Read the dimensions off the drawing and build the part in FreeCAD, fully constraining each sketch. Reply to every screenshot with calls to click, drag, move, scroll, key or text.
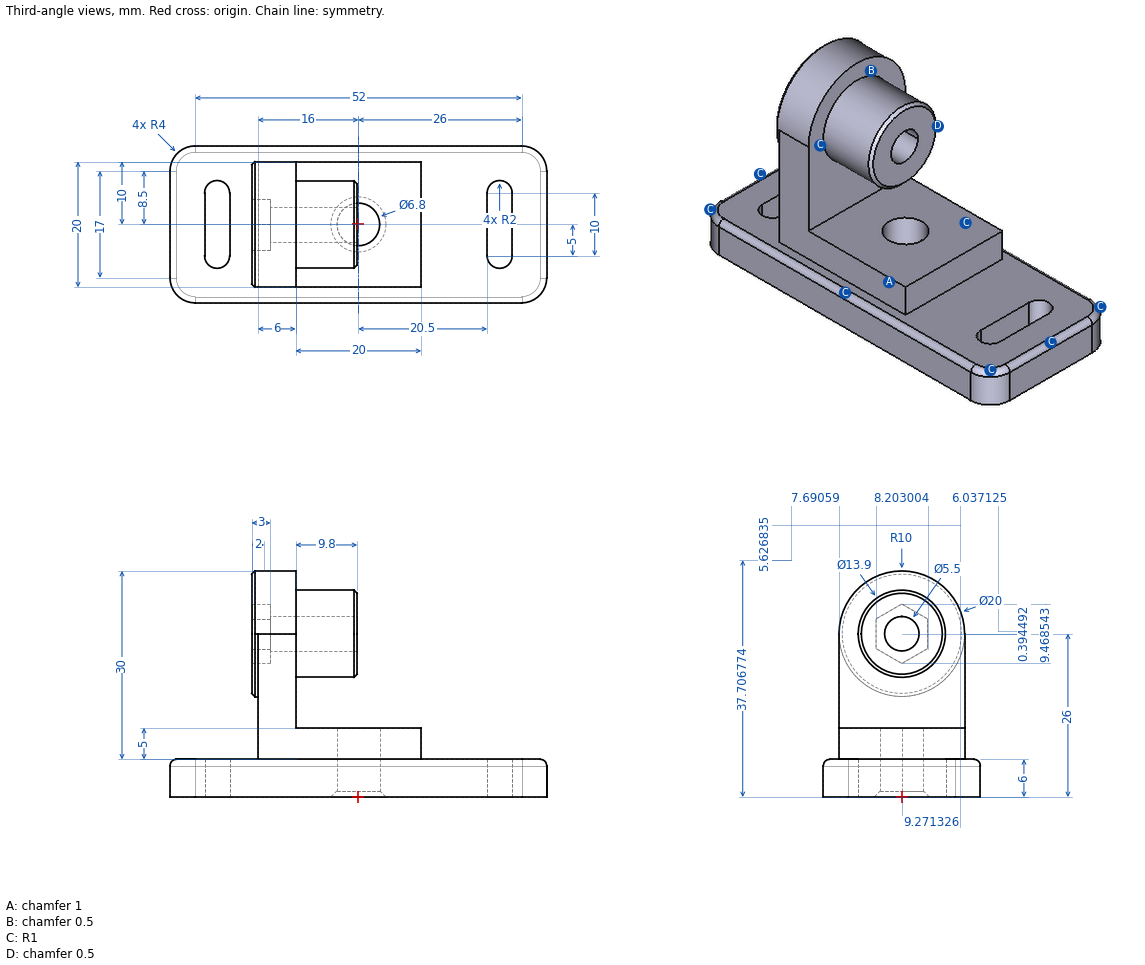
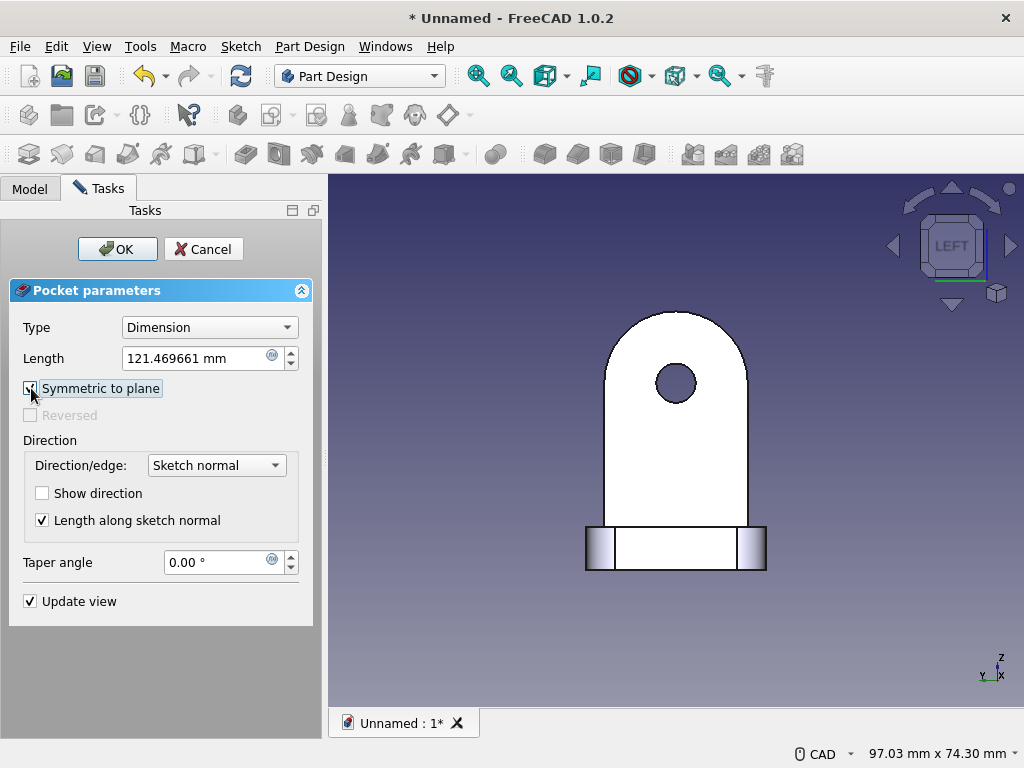
click(118, 249)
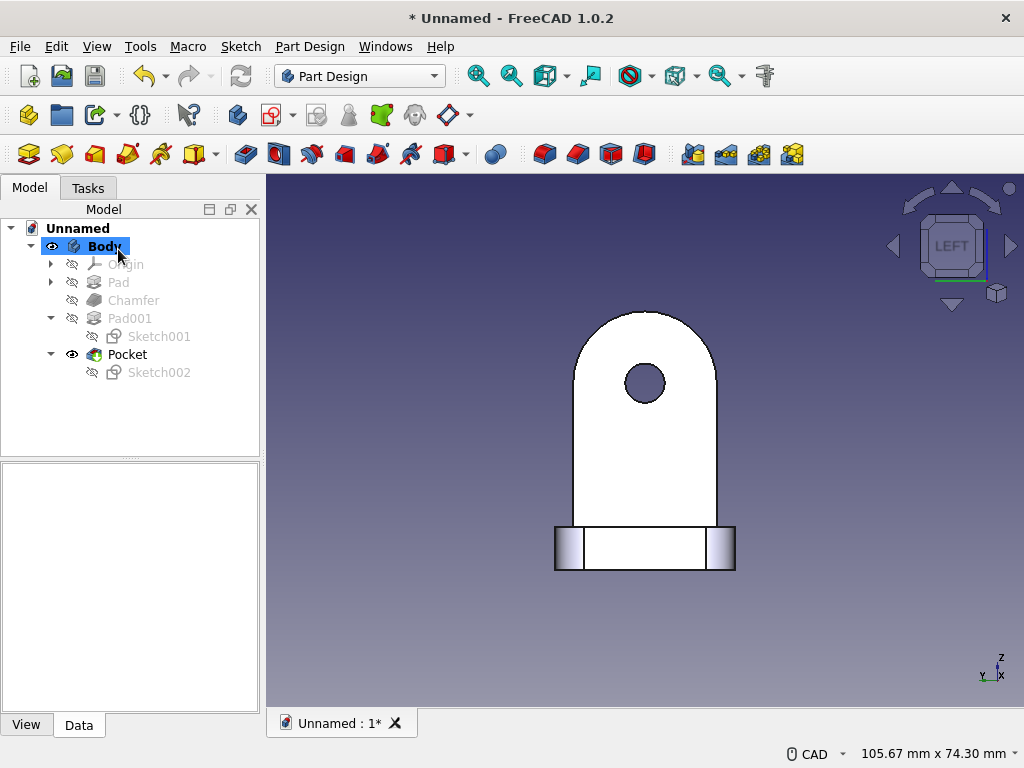
click(625, 449)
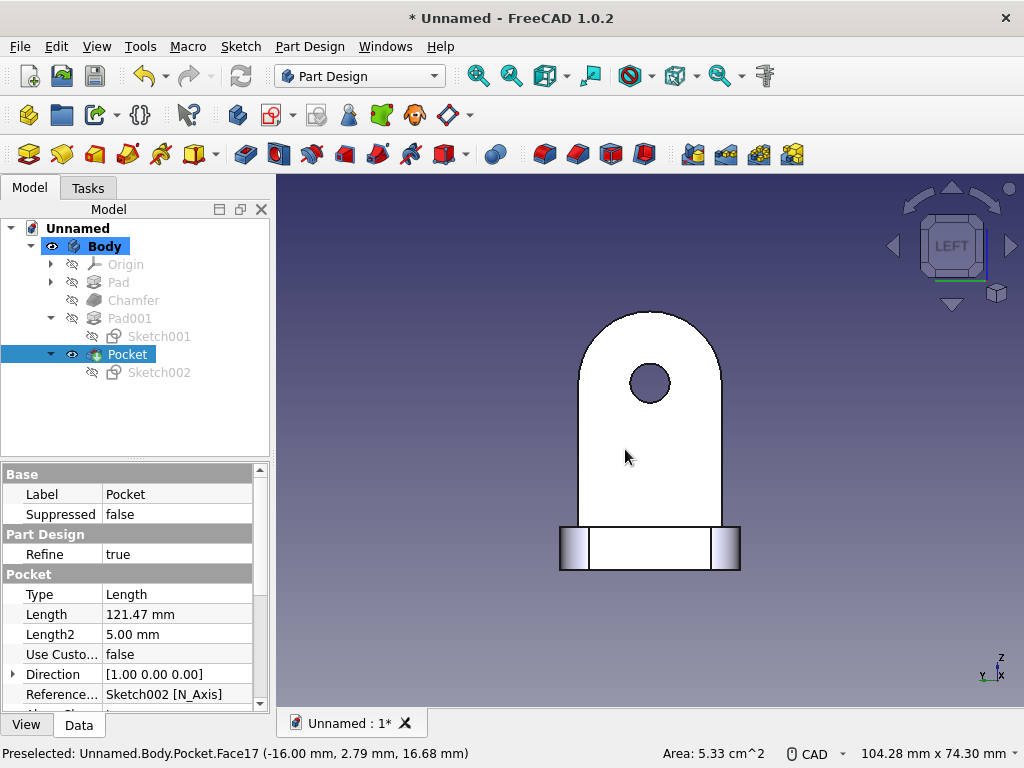
click(270, 116)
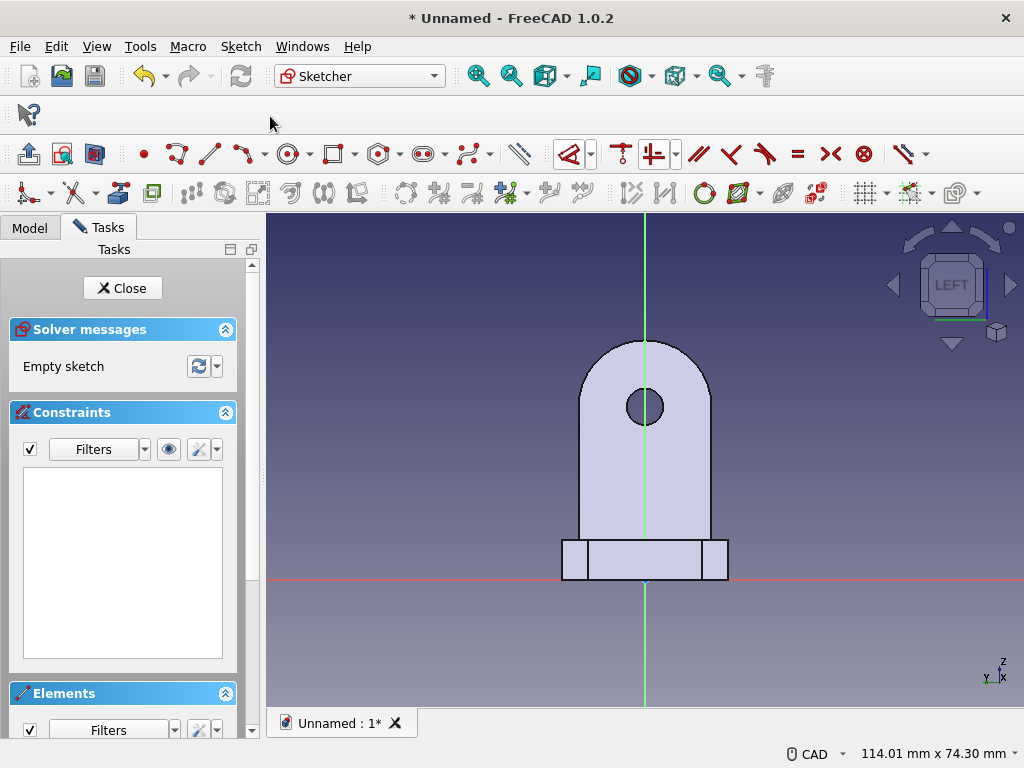
click(95, 154)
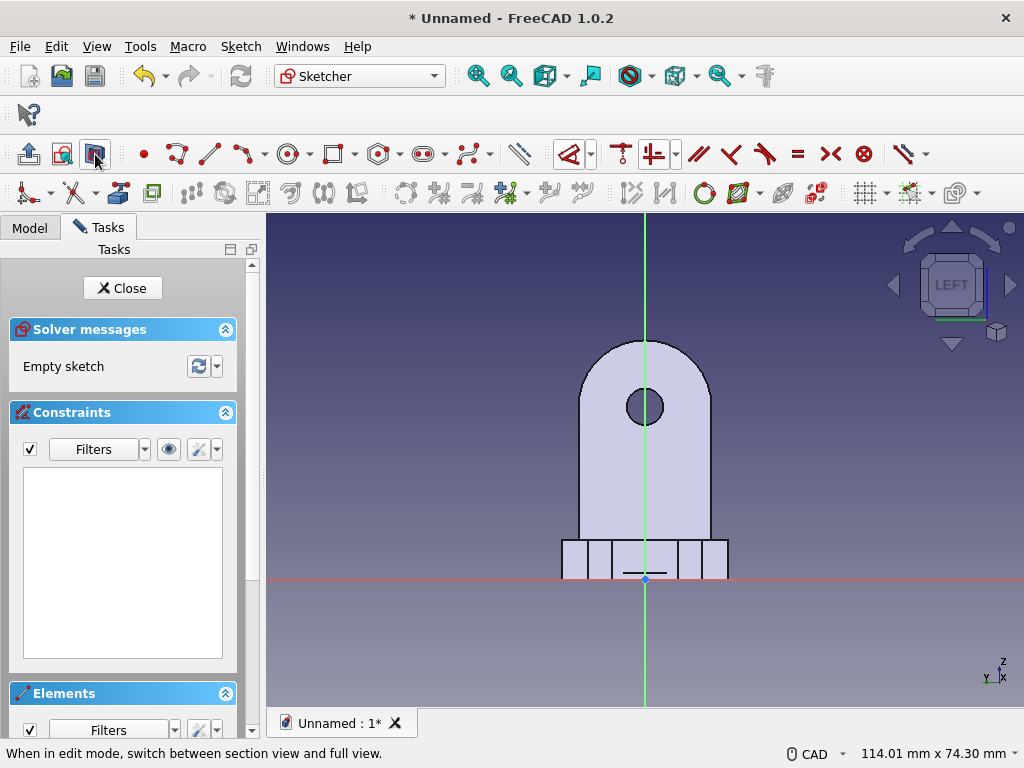
click(288, 154)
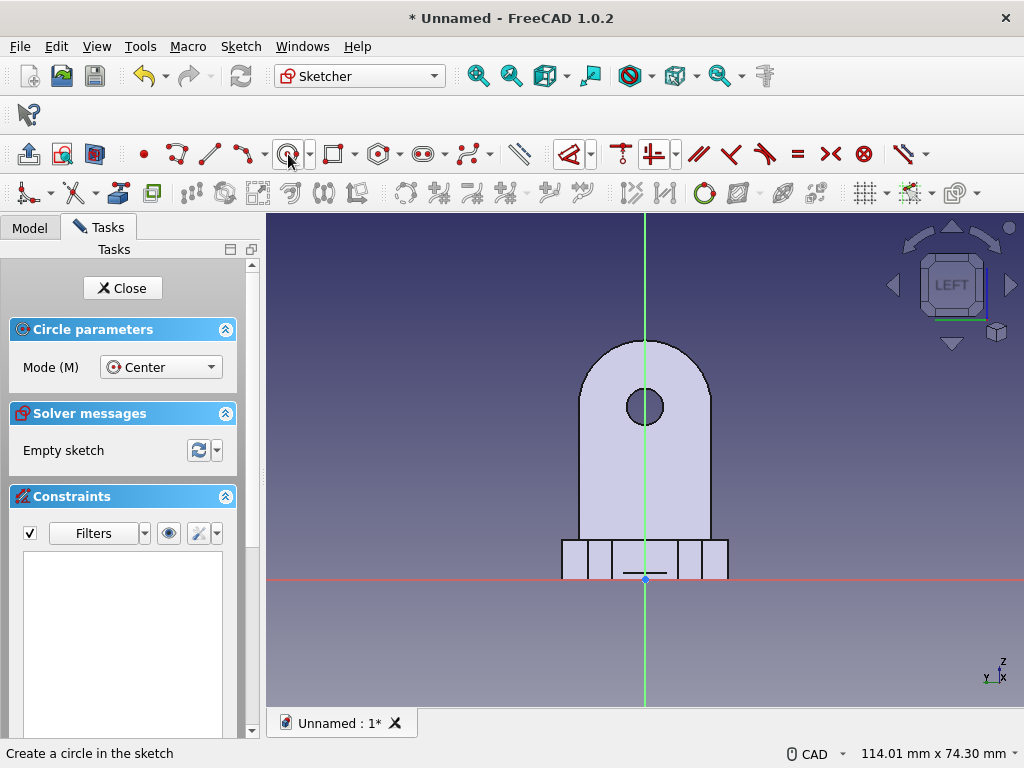
click(645, 407)
move(692, 360)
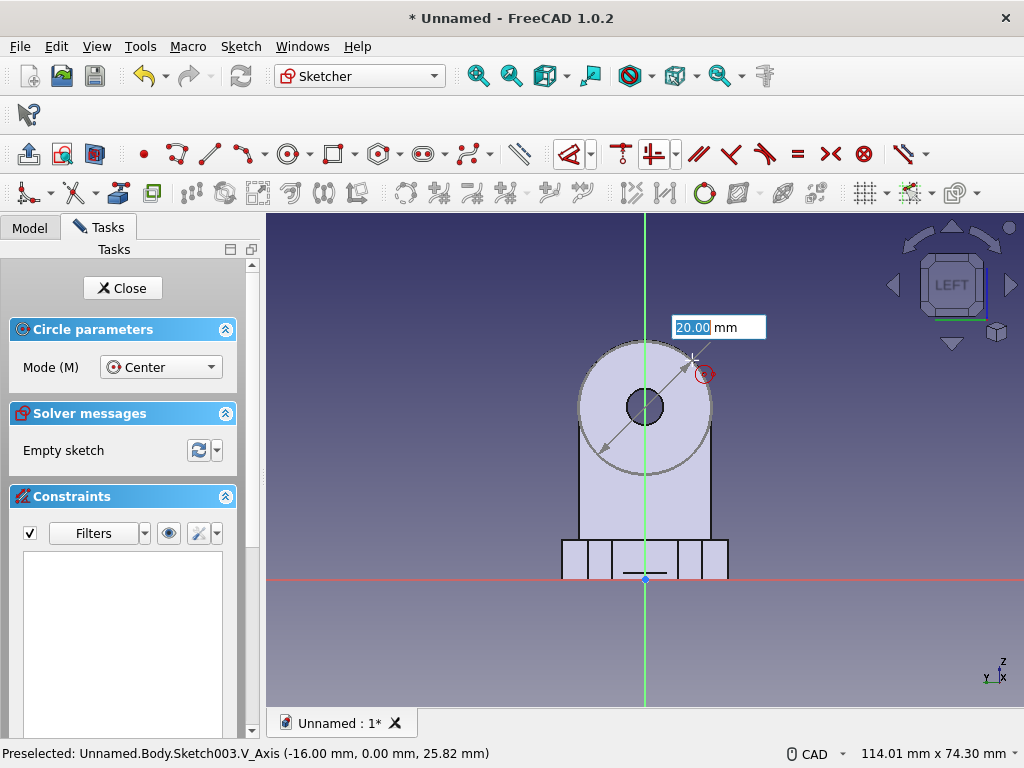
text(20)
key(Return)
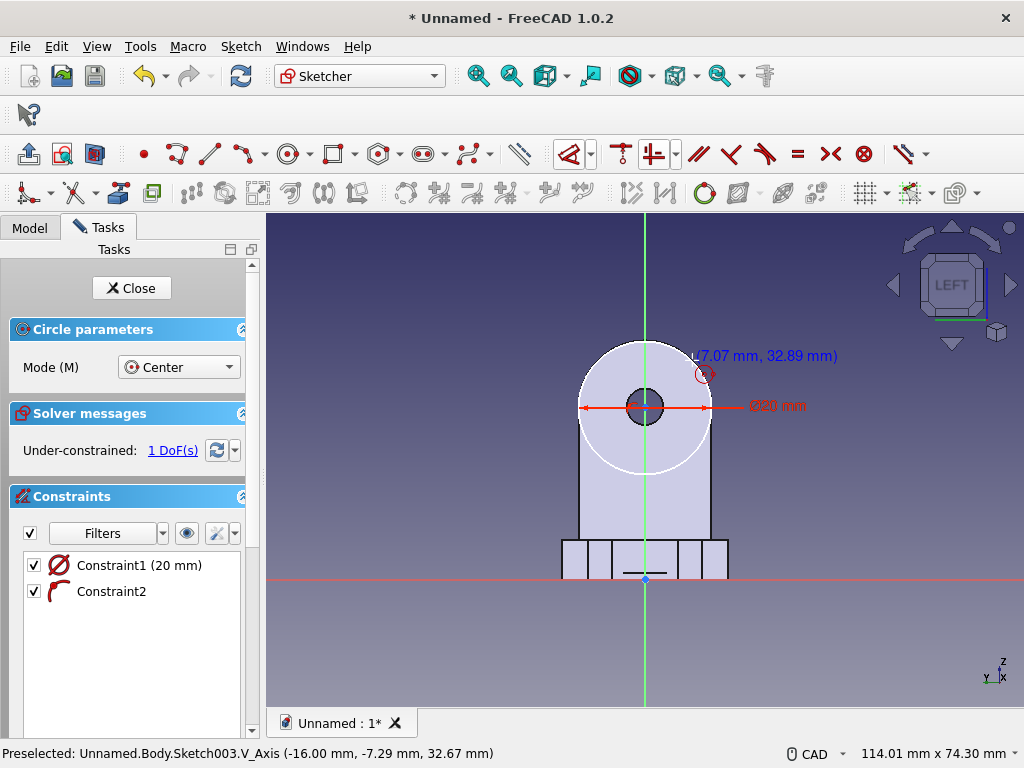
scroll(645, 407, up, 2)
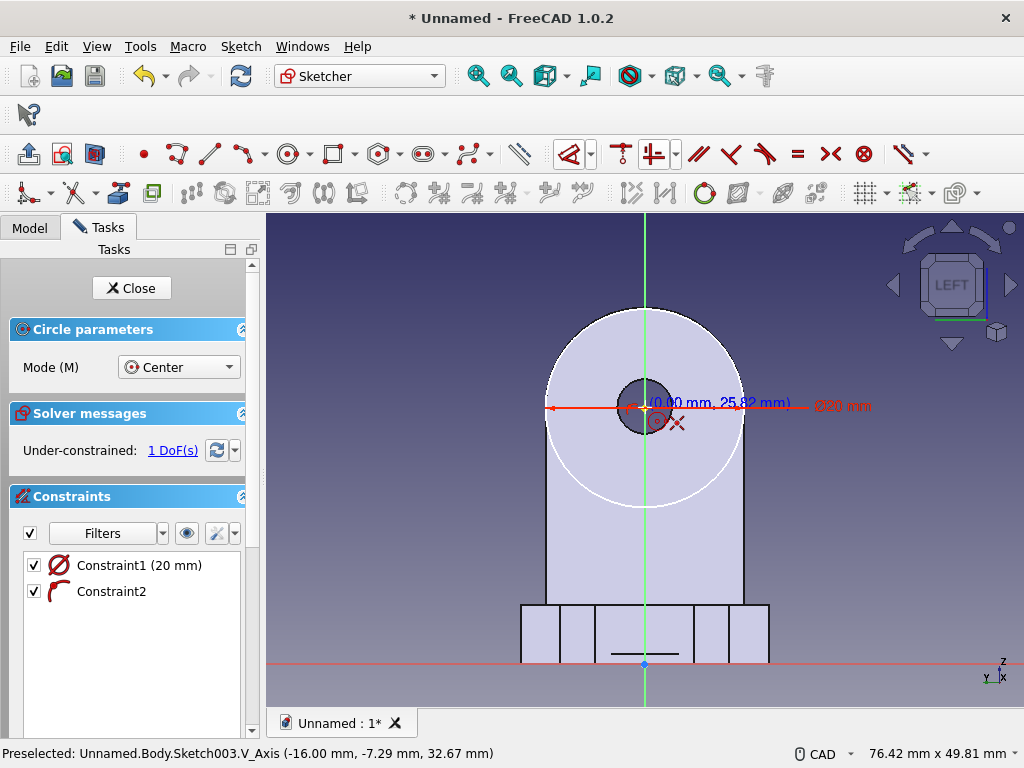
click(645, 408)
move(664, 387)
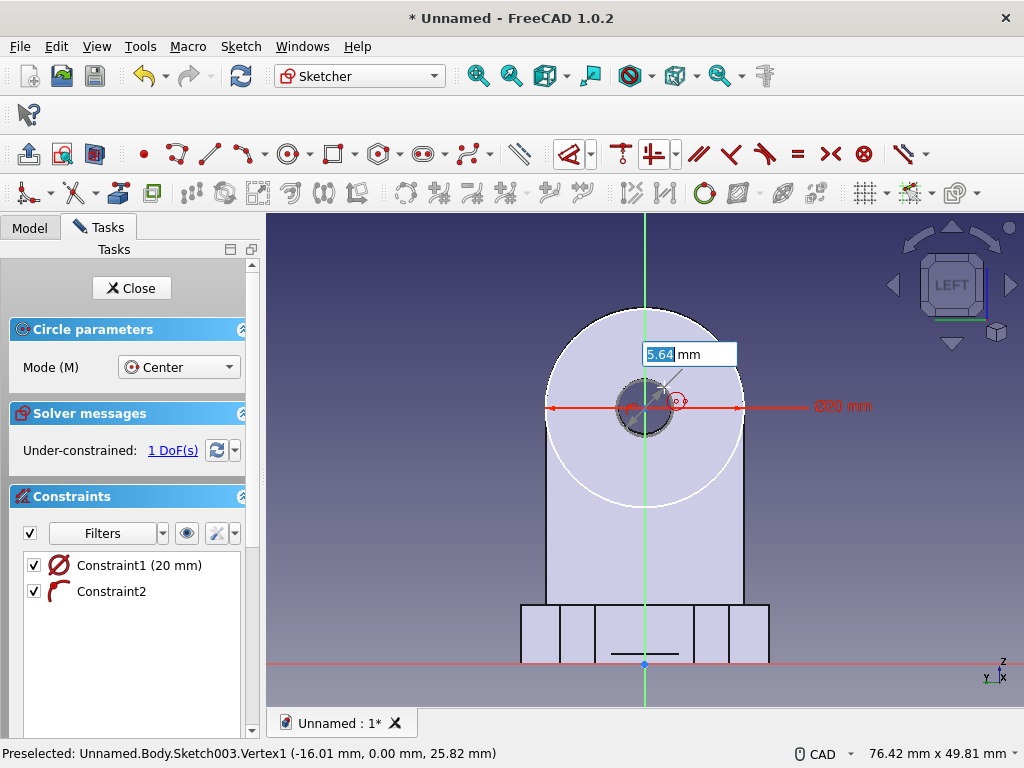
text(5.5)
key(Return)
key(Escape)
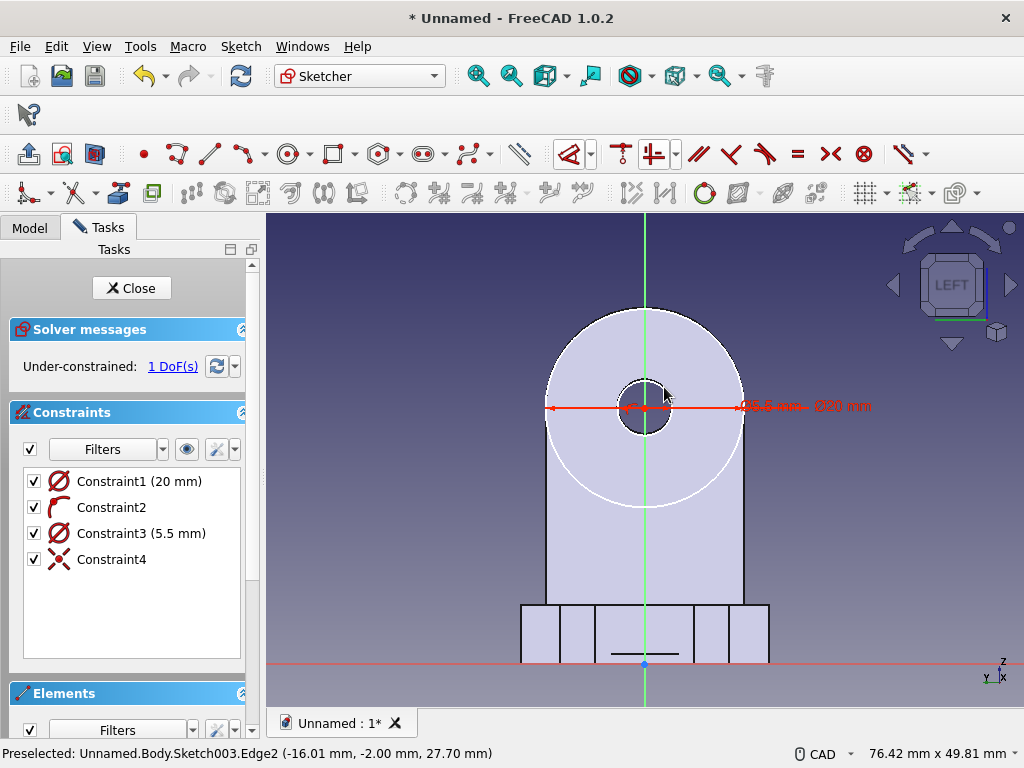
click(645, 408)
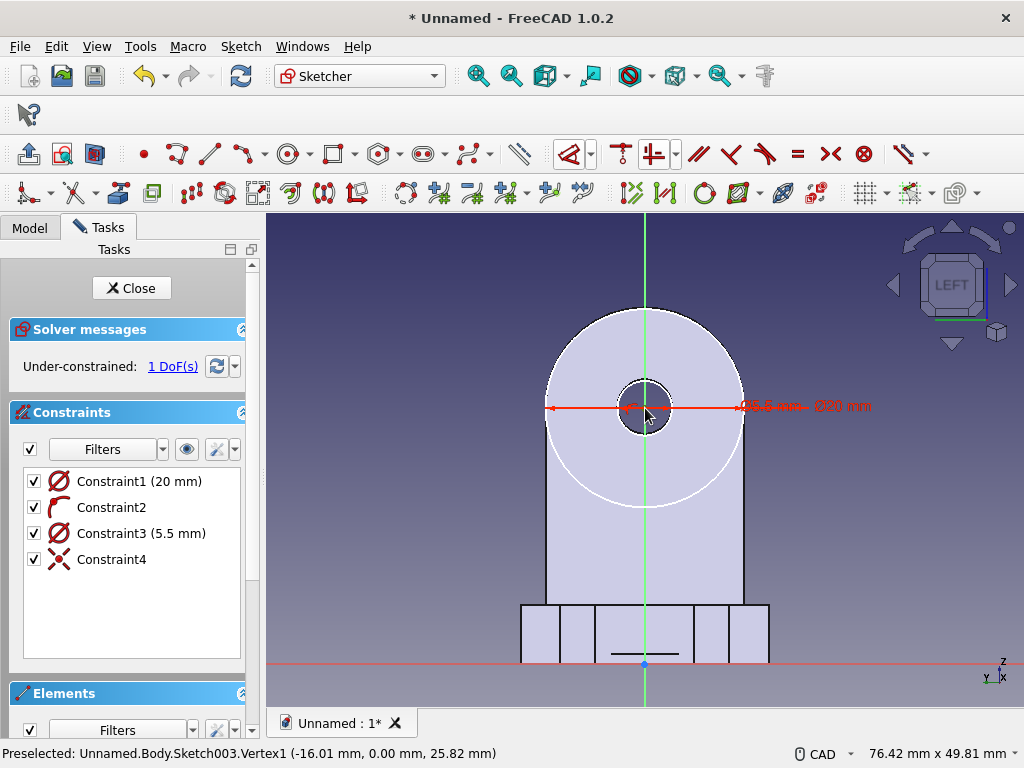
click(590, 154)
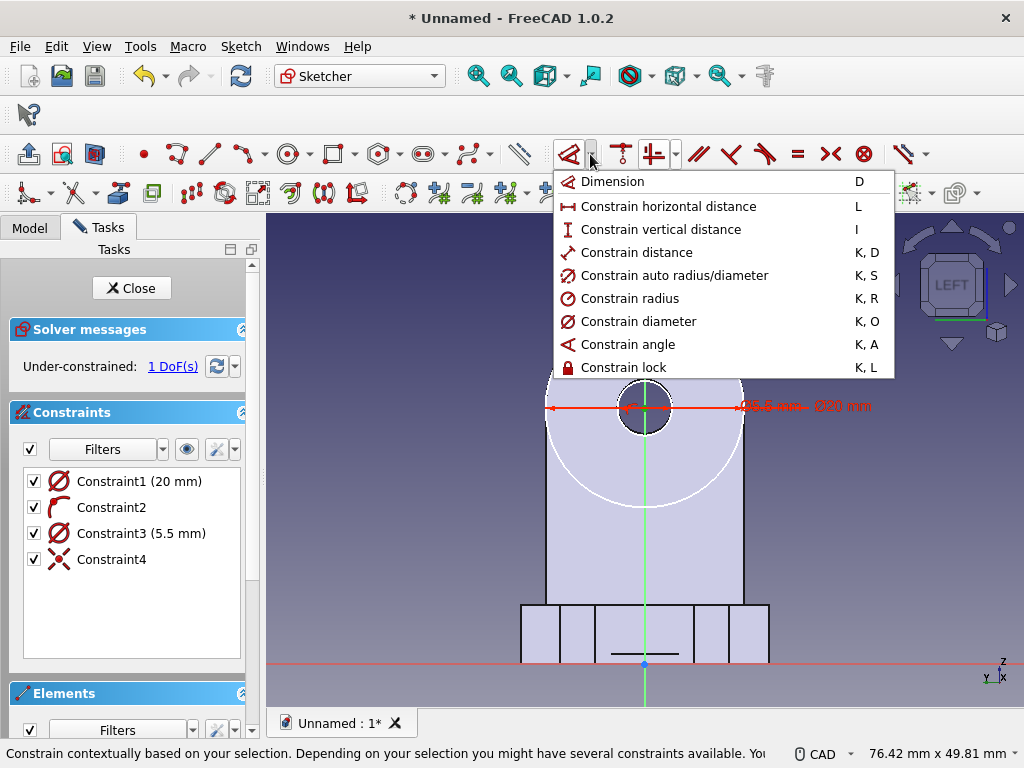
click(724, 230)